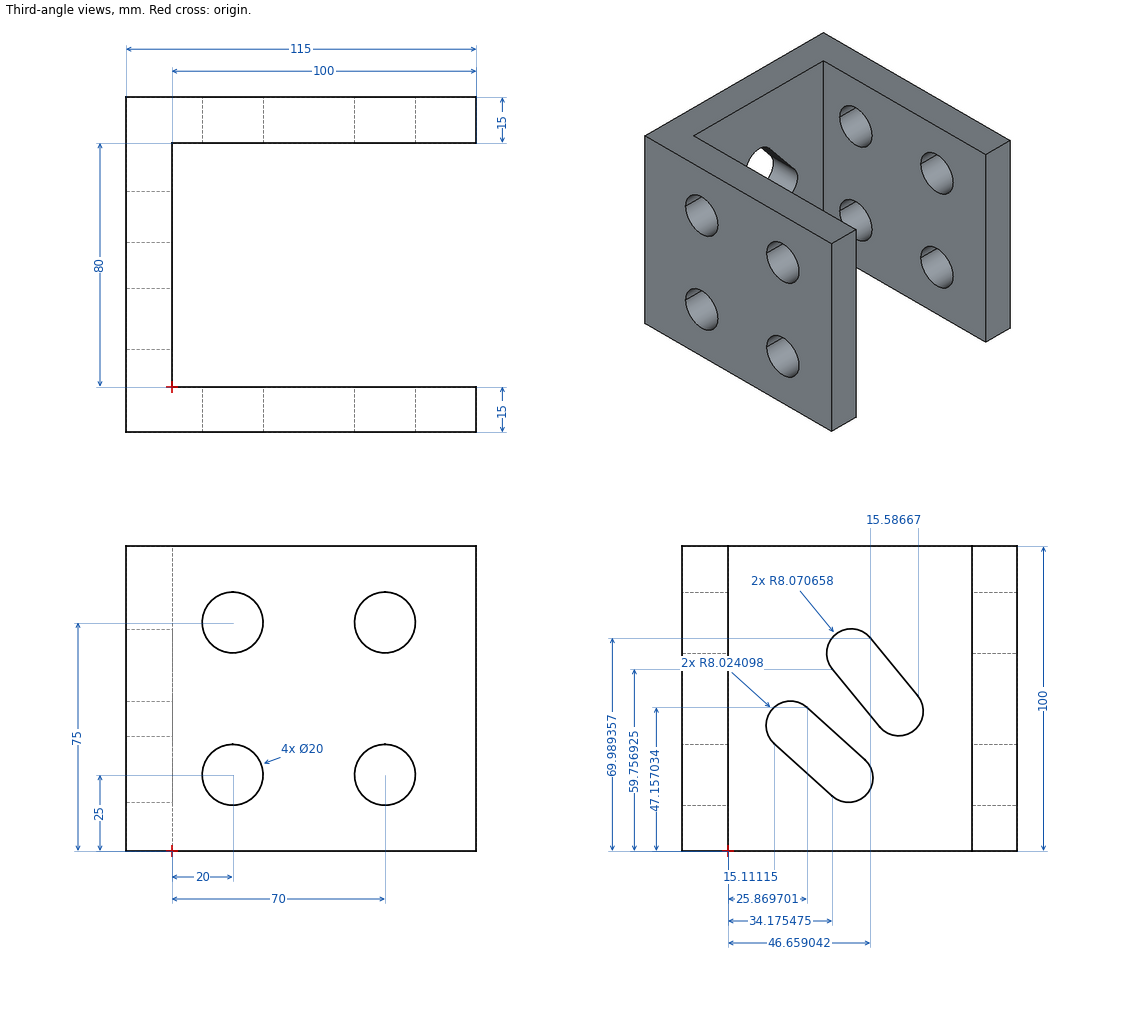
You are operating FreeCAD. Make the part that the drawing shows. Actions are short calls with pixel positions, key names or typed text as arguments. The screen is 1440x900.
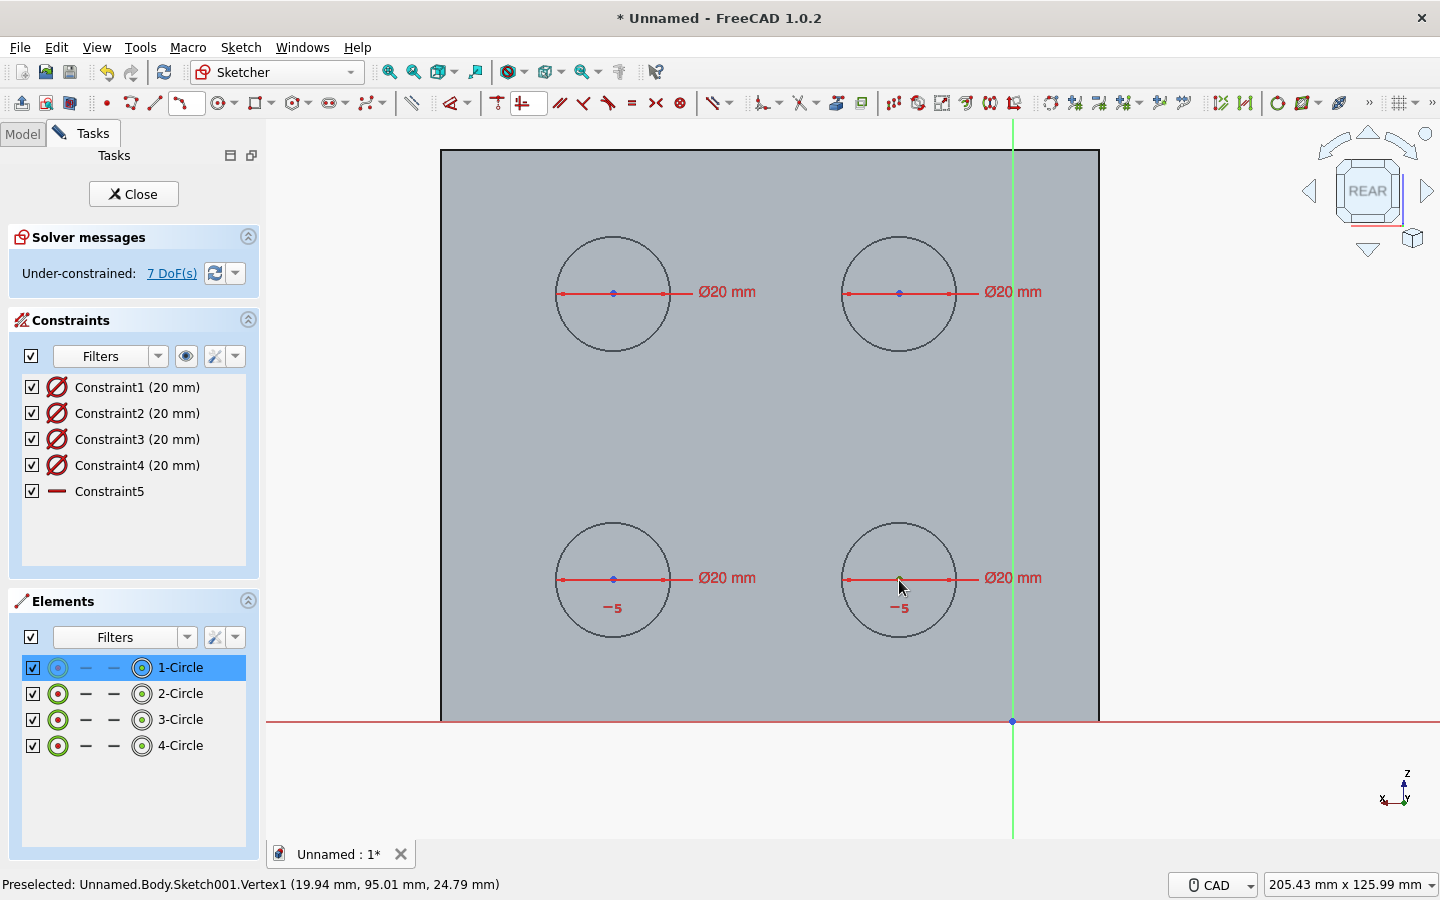
click(899, 294)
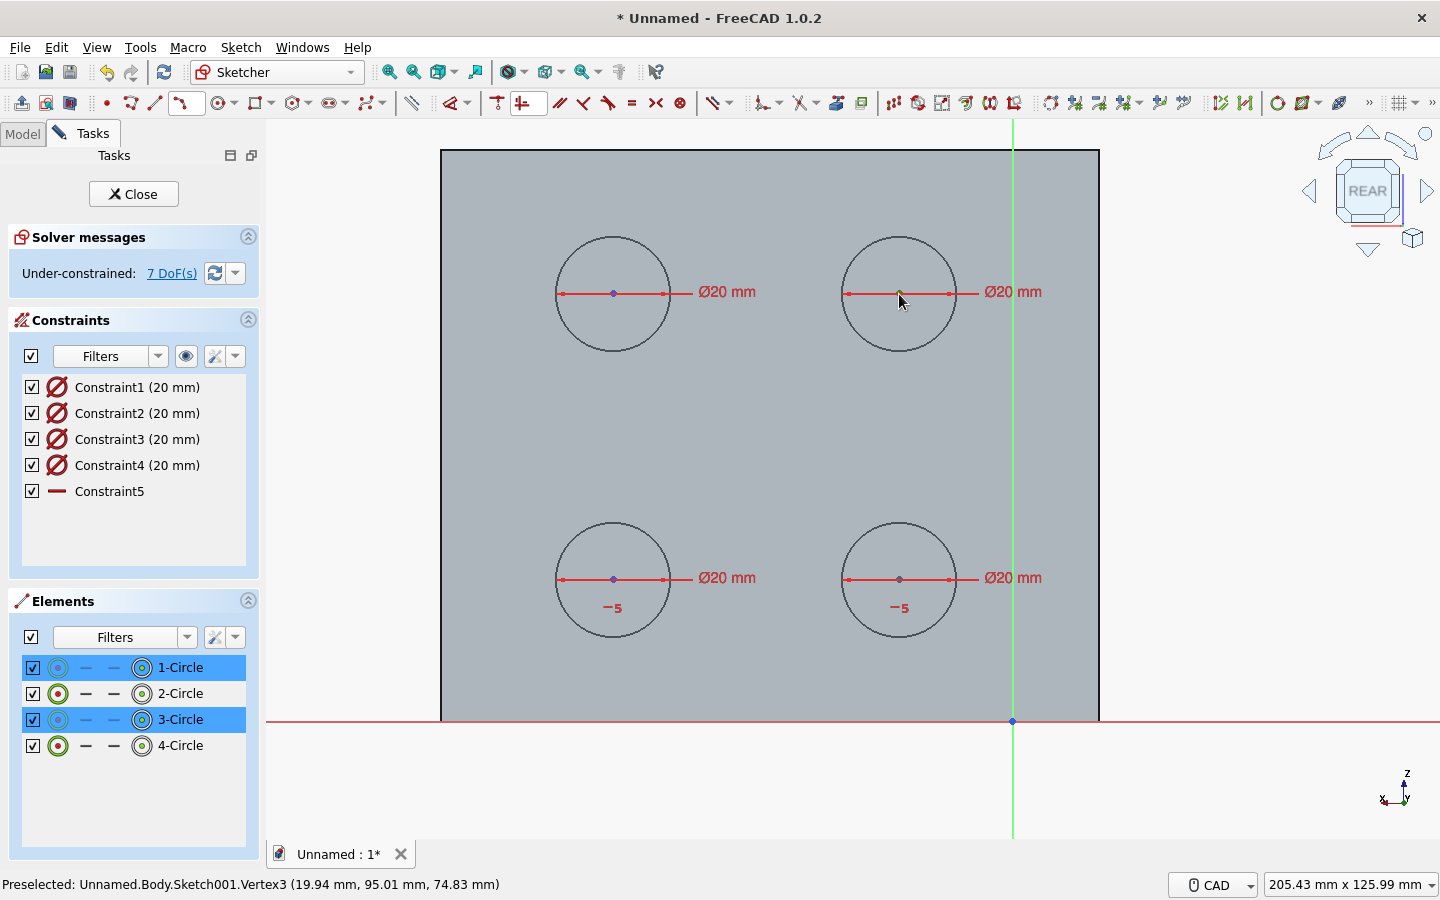
key(v)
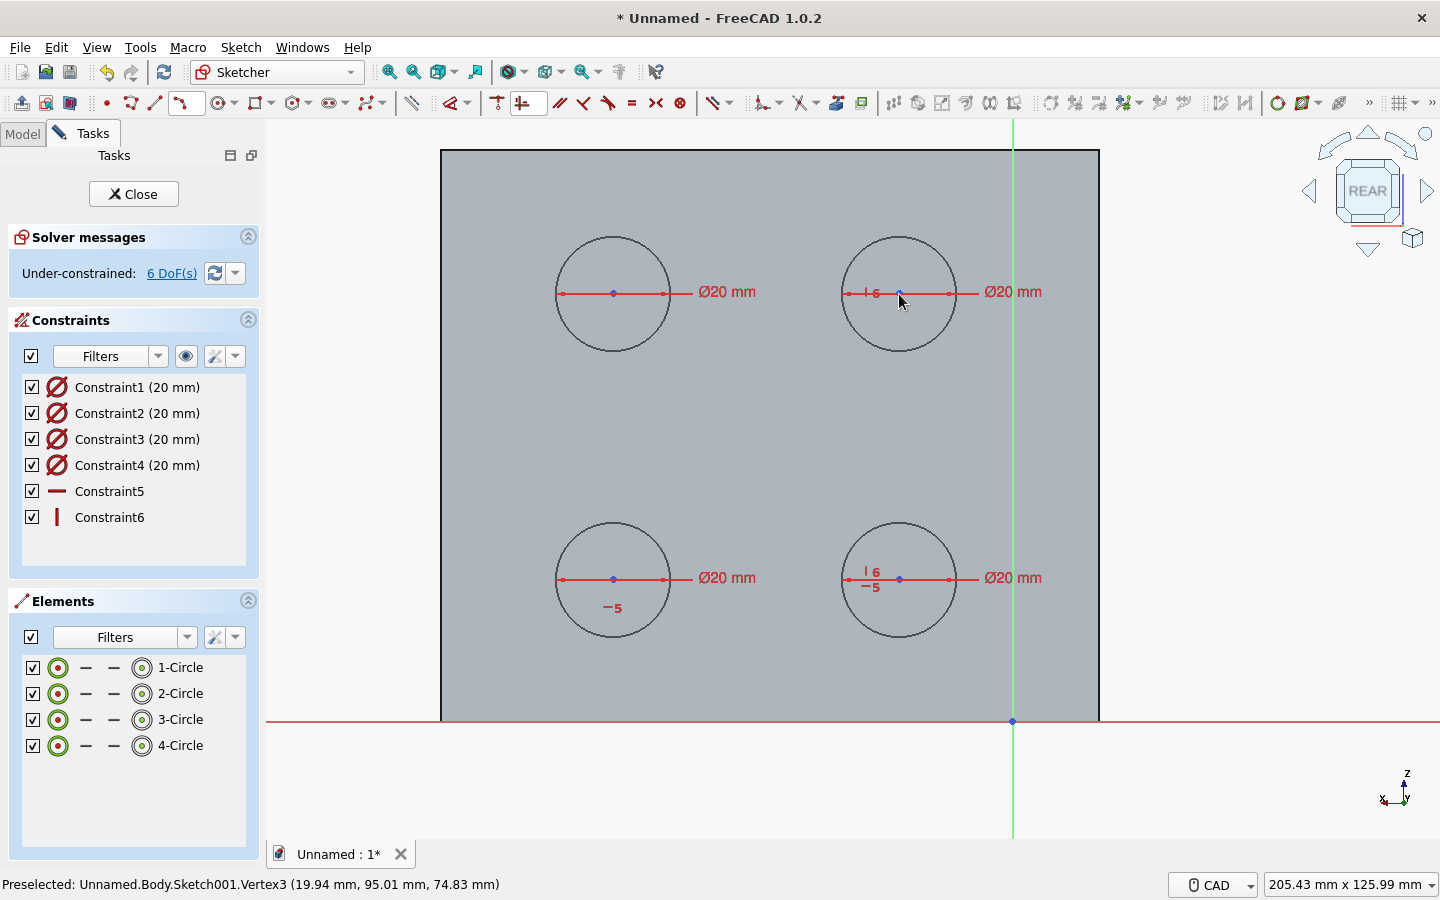
click(613, 580)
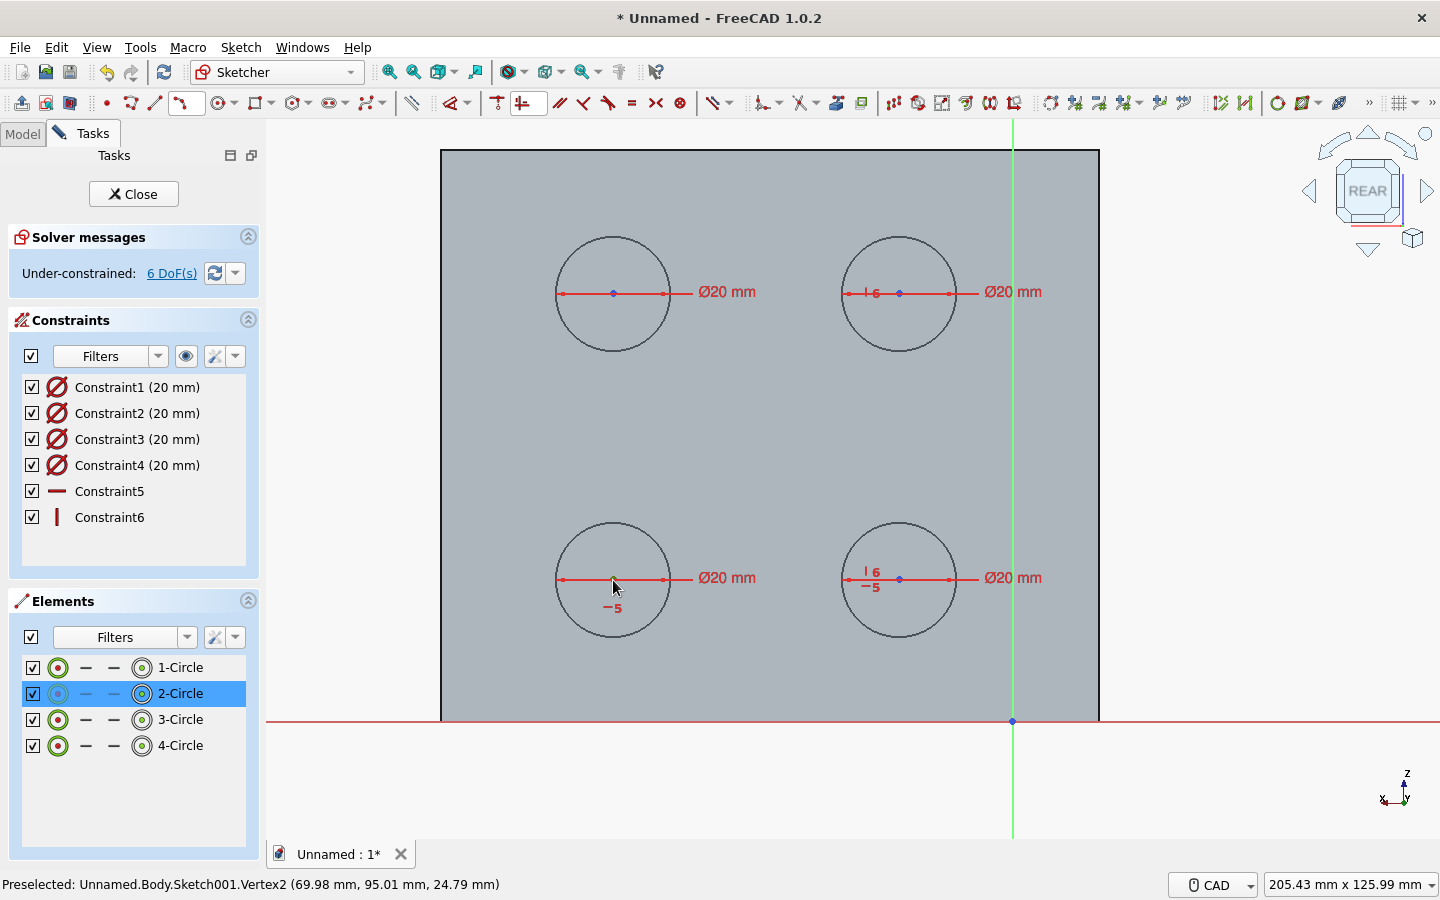
click(613, 294)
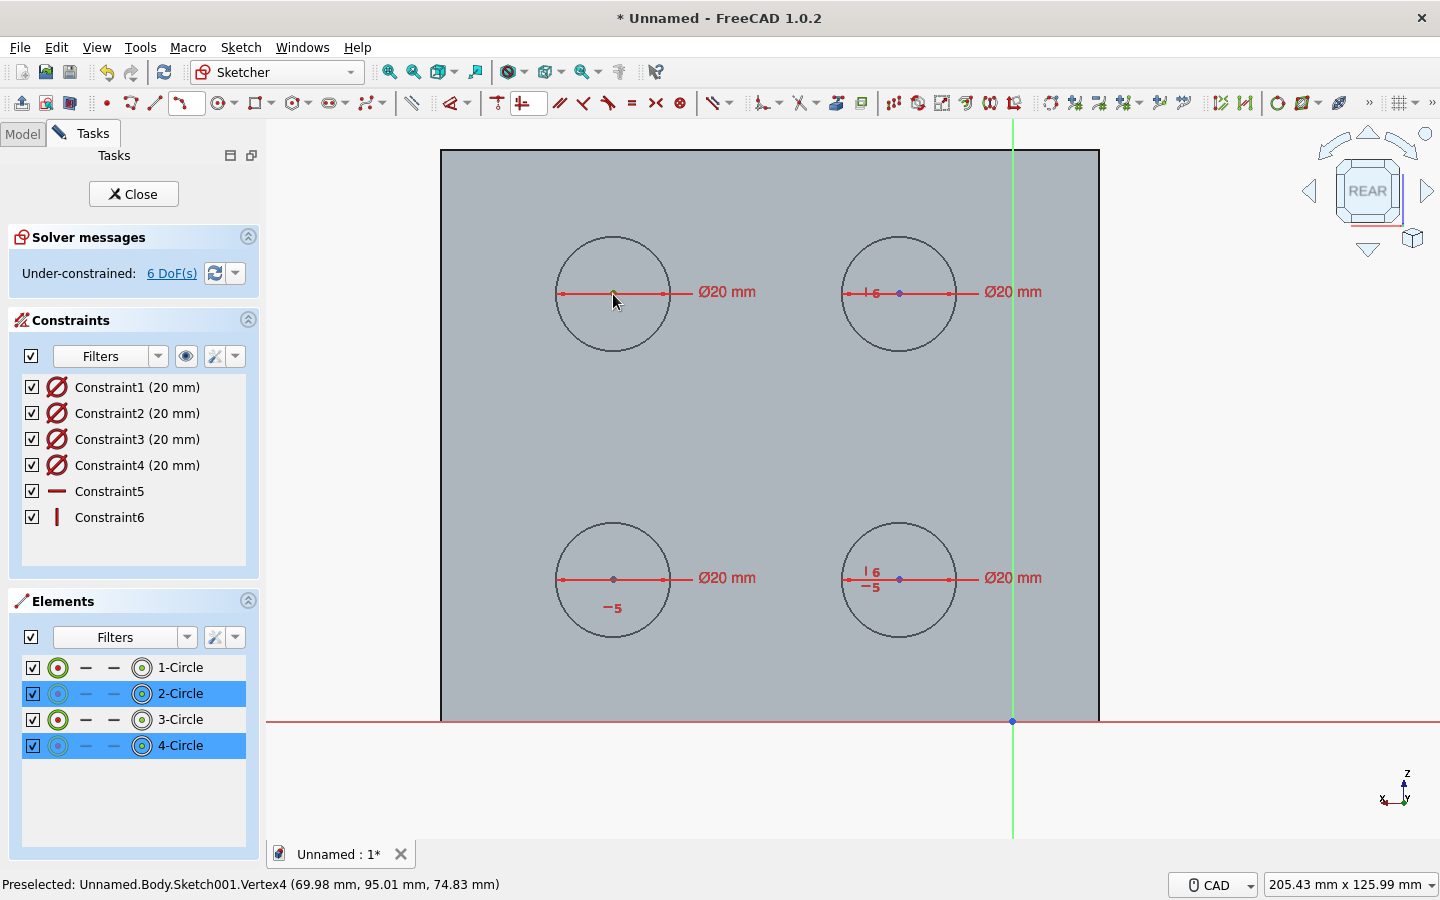
key(v)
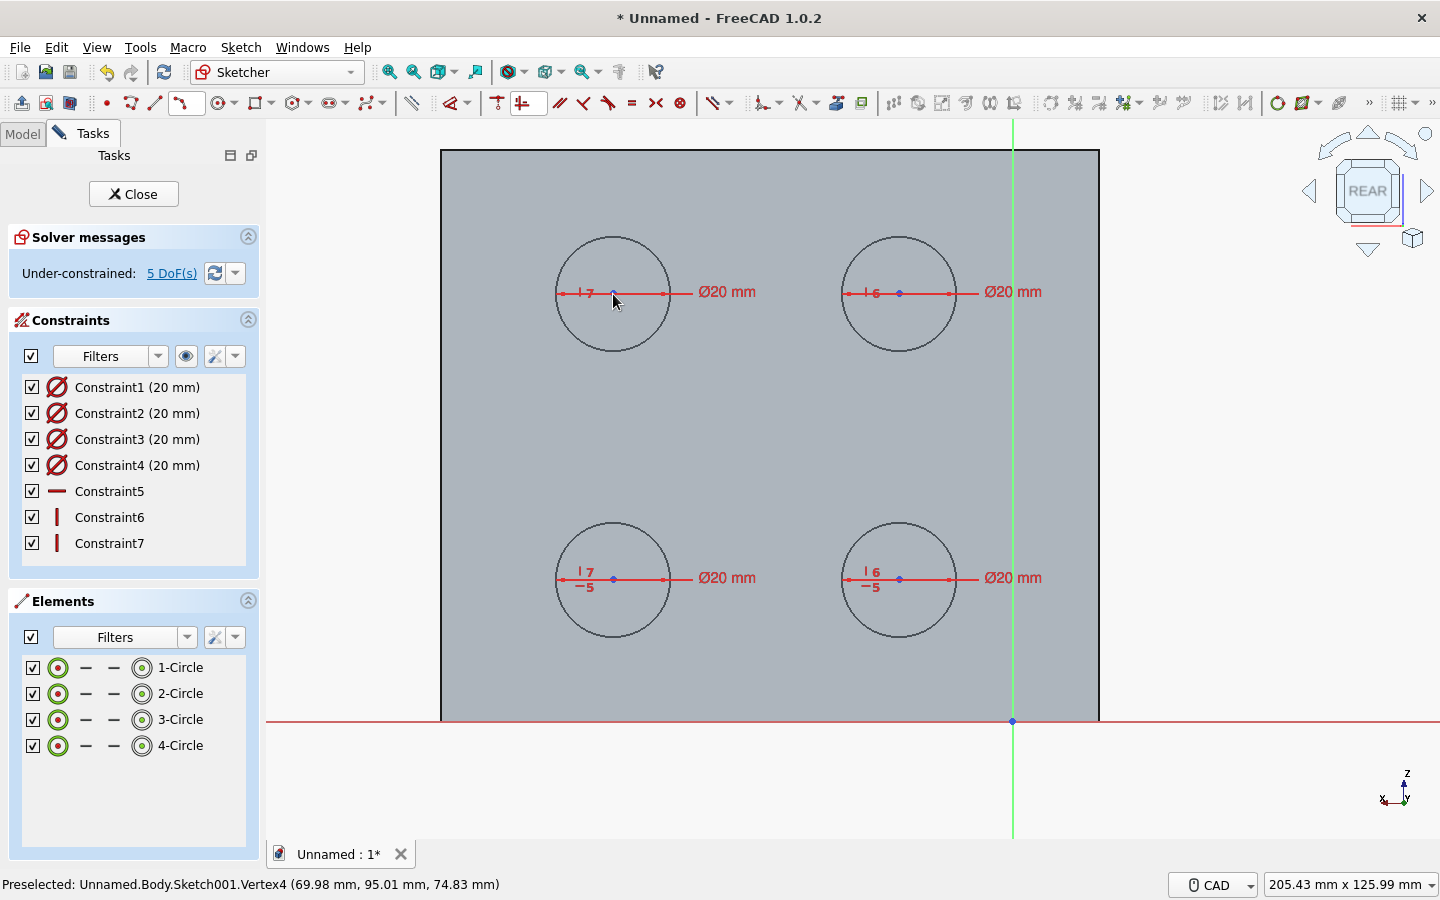
click(899, 294)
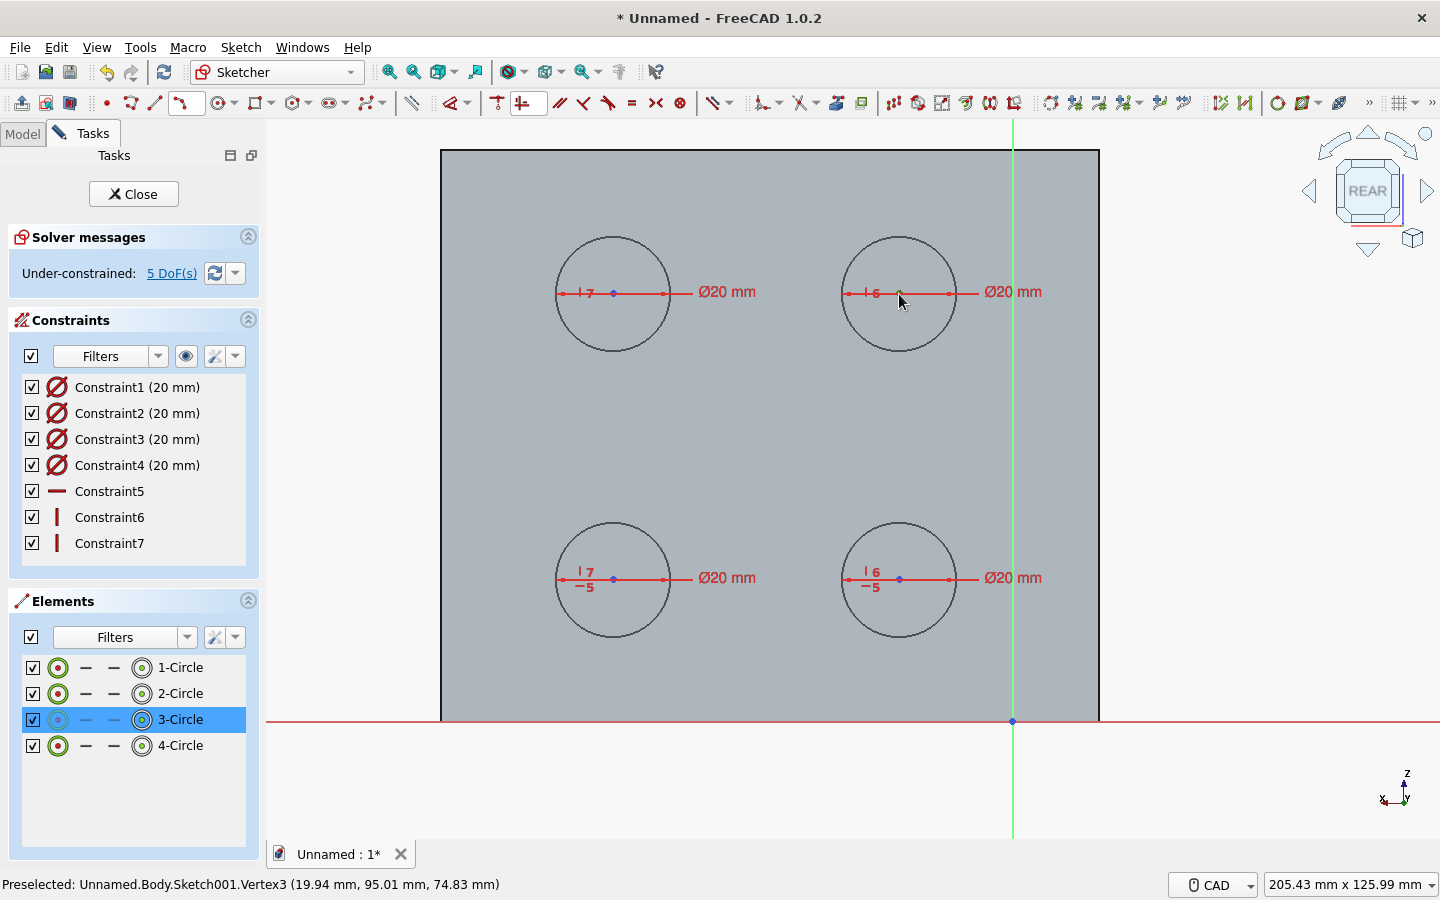
click(613, 294)